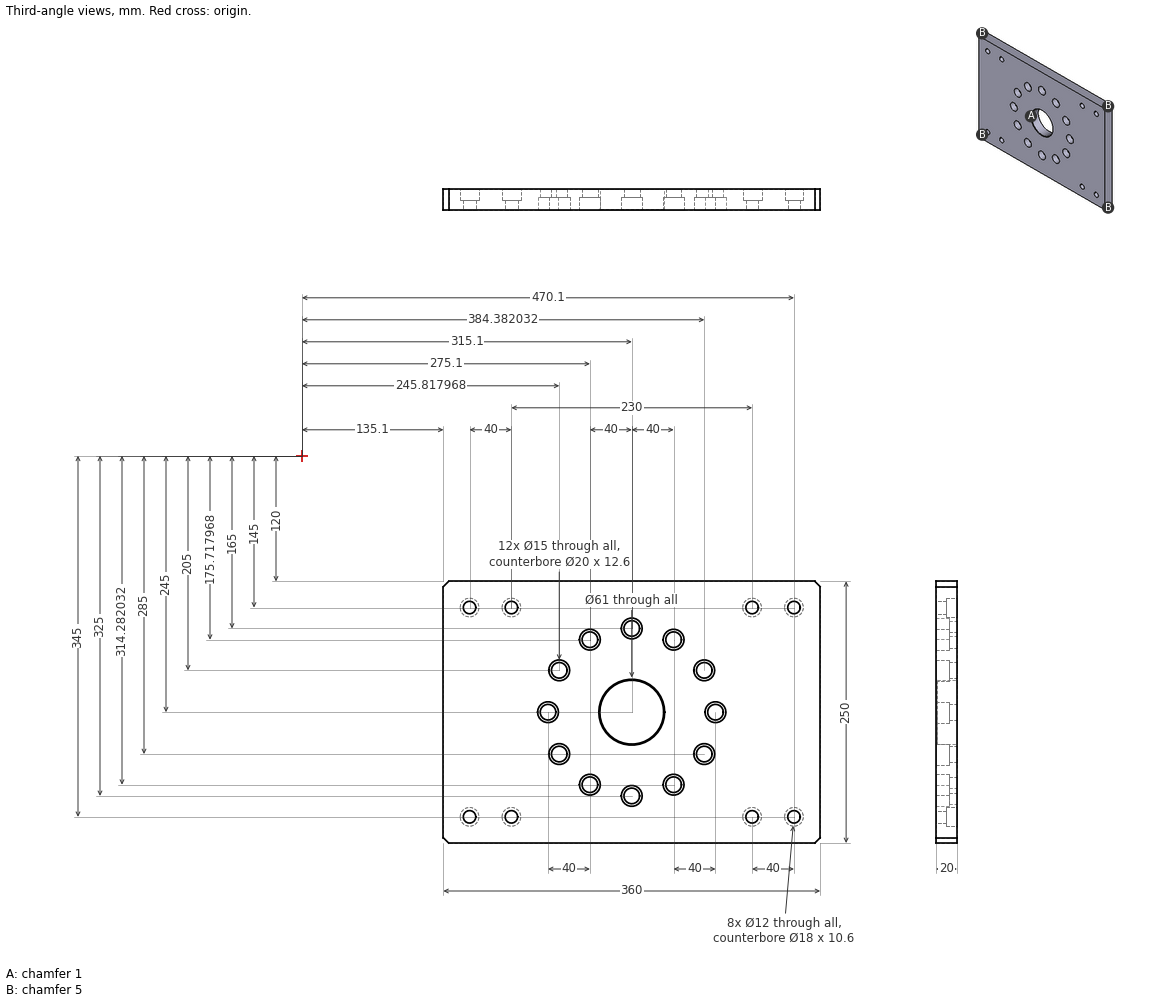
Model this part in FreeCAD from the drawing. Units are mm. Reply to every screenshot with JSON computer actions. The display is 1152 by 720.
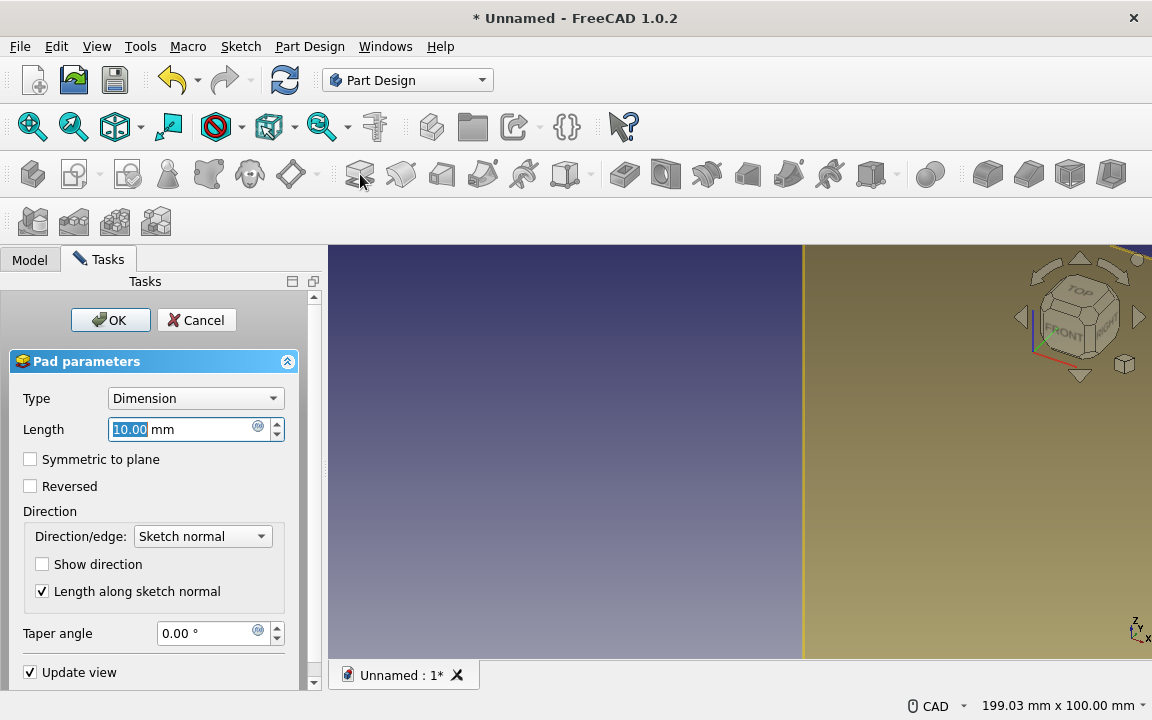
{"action": "type", "text": "20"}
{"action": "key", "text": "Tab"}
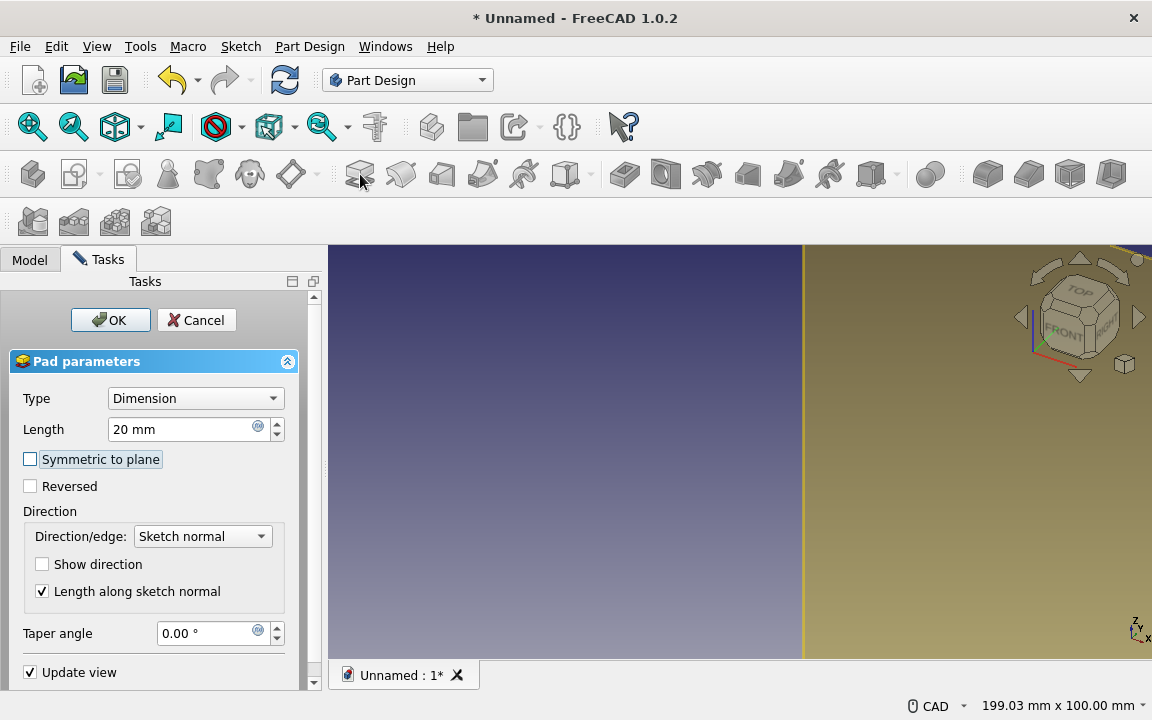
{"action": "left_click", "coordinate": [31, 486]}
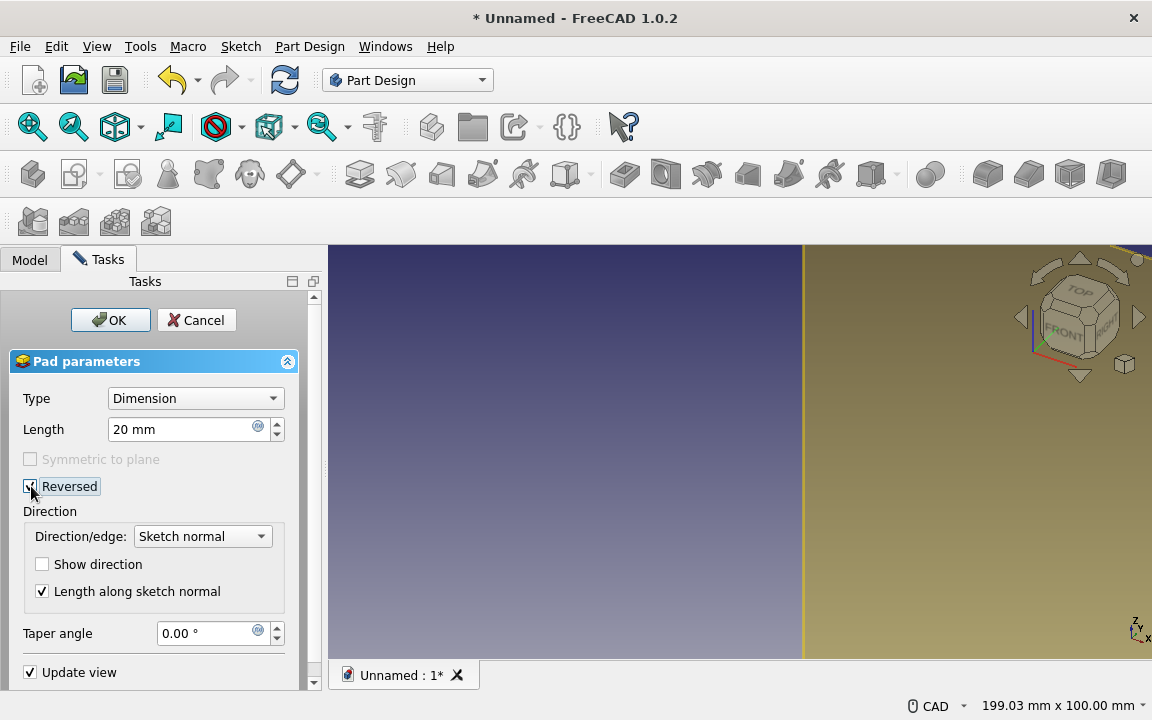
{"action": "left_click", "coordinate": [111, 320]}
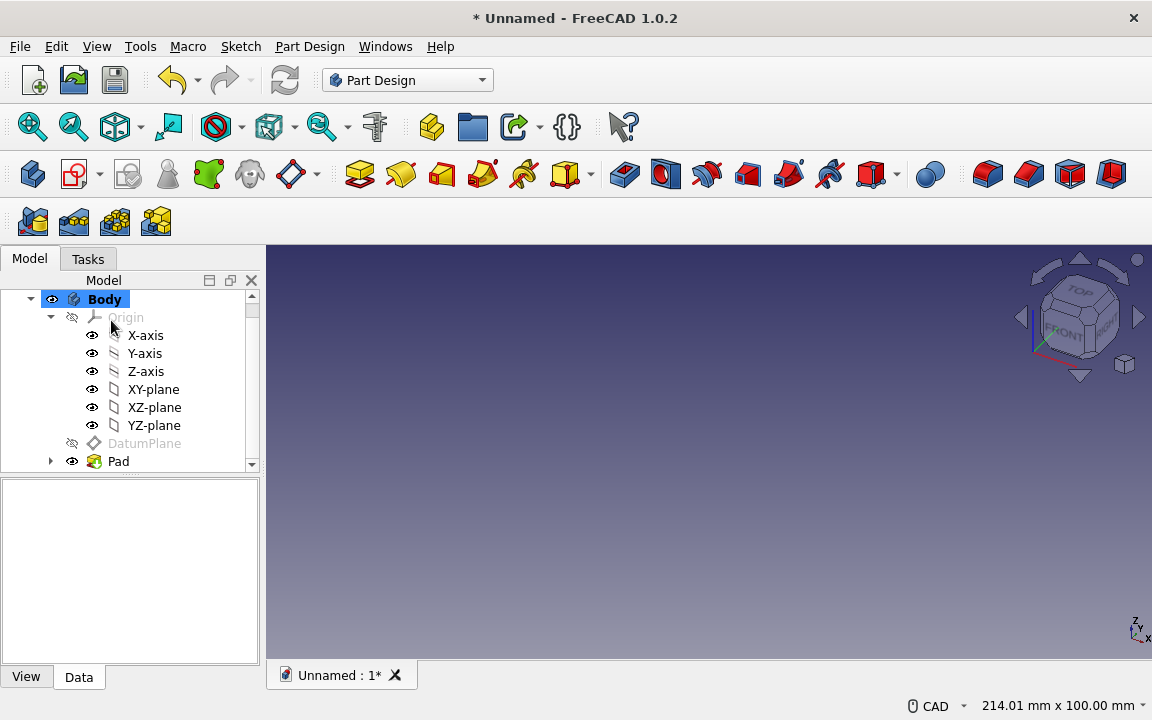
{"action": "left_click", "coordinate": [33, 128]}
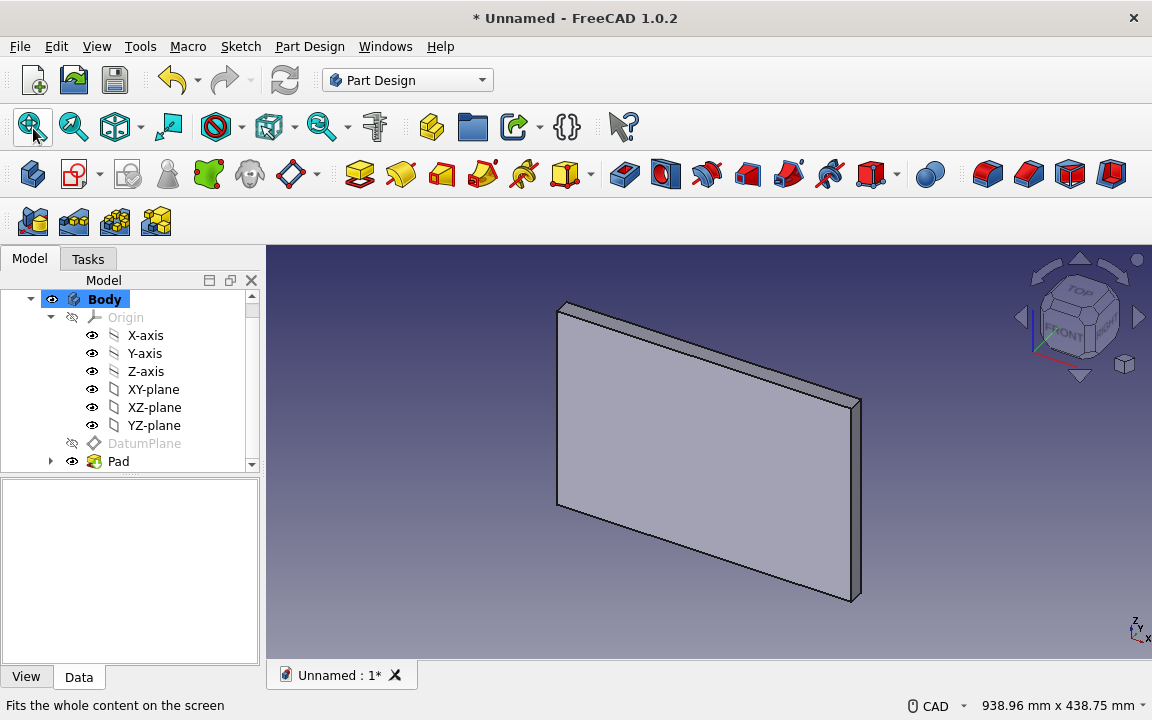
{"action": "key", "text": "4"}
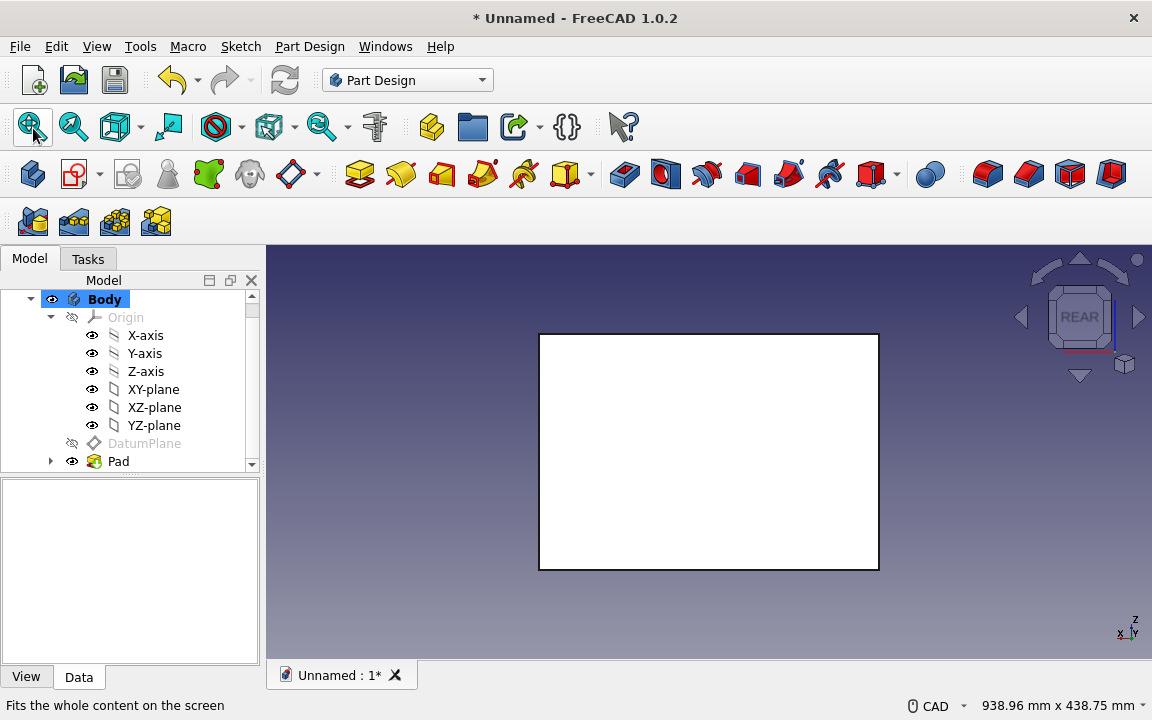
{"action": "left_click", "coordinate": [660, 451]}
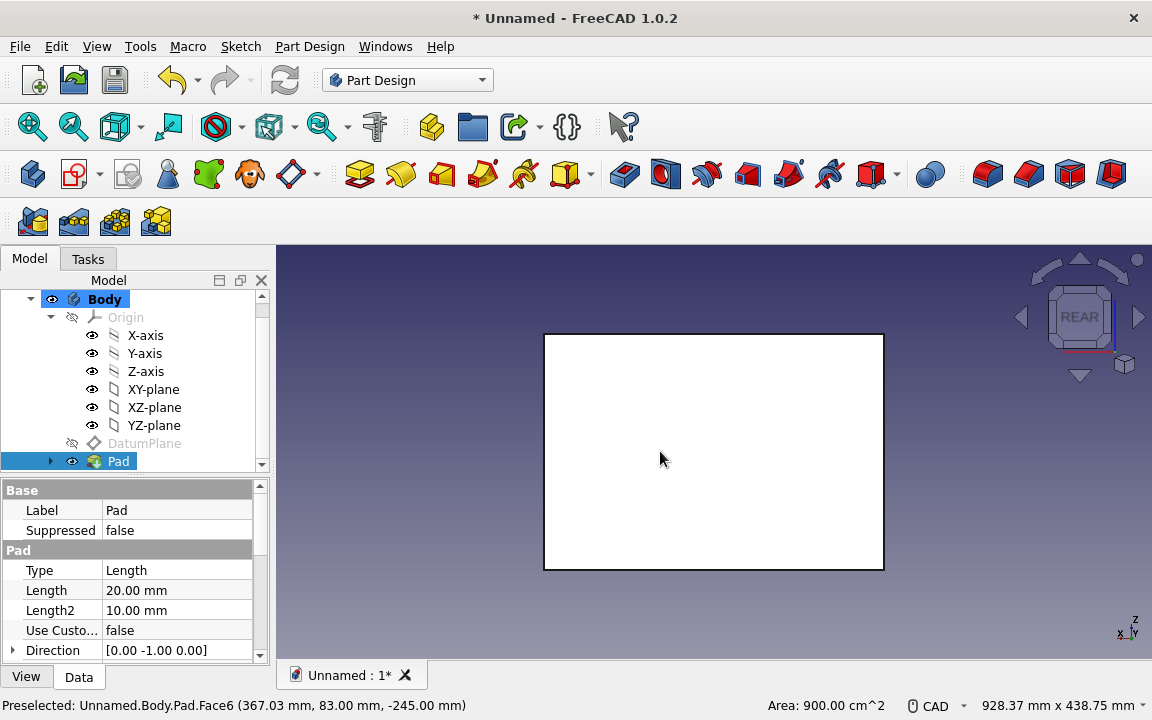
{"action": "left_click", "coordinate": [74, 174]}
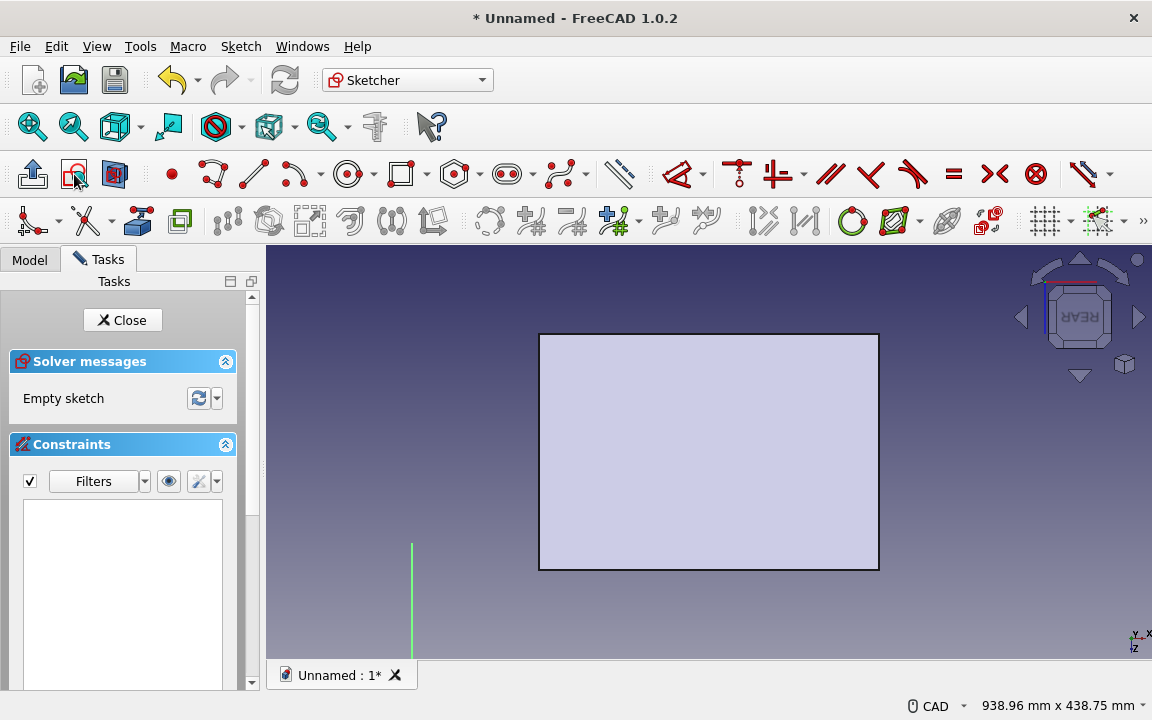
{"action": "scroll", "coordinate": [649, 319], "scroll_direction": "down", "scroll_amount": 2}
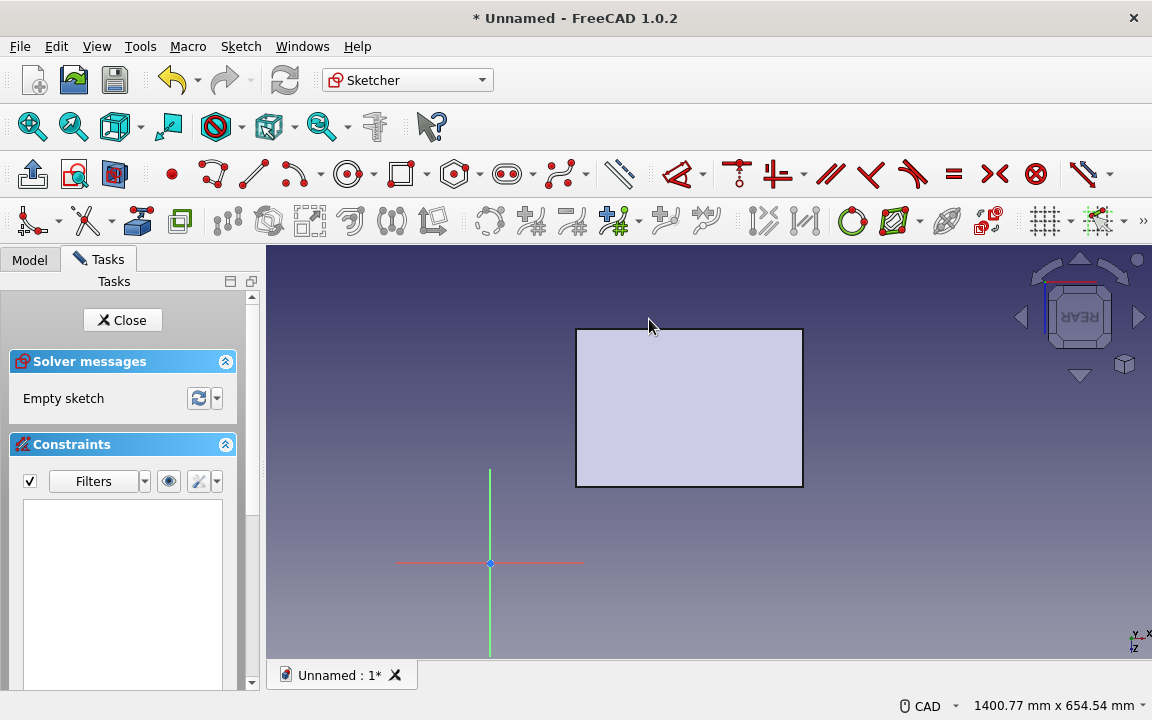
{"action": "left_click", "coordinate": [348, 174]}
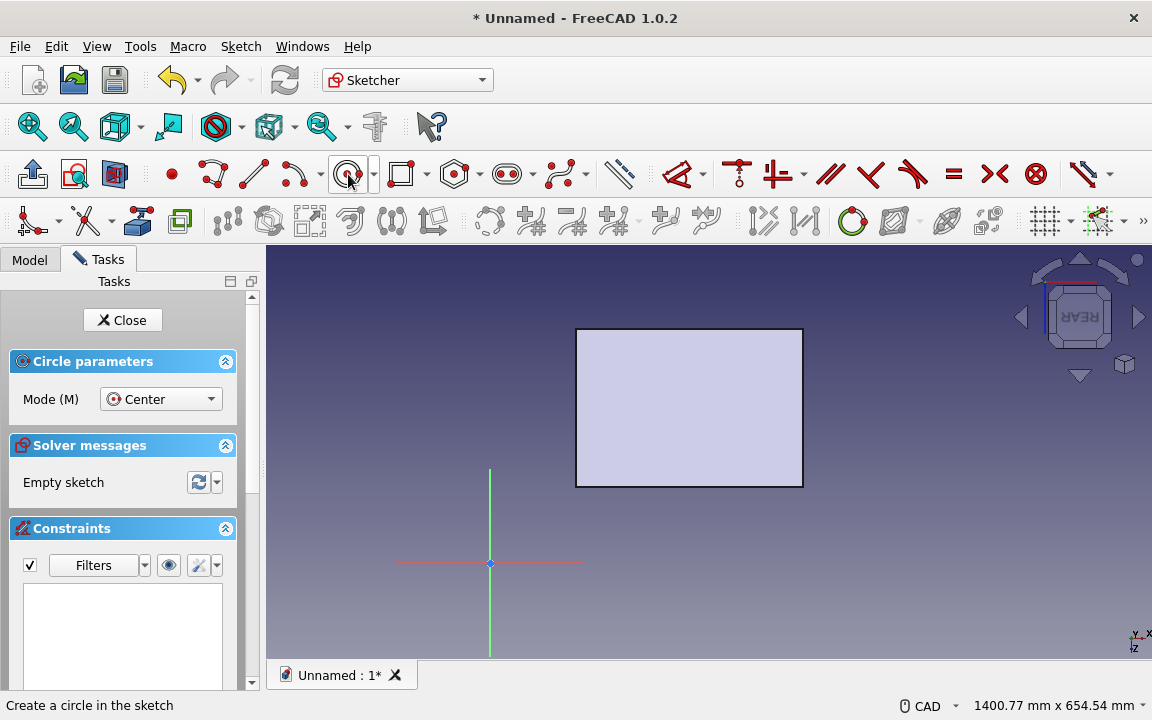
{"action": "scroll", "coordinate": [787, 345], "scroll_direction": "up", "scroll_amount": 9}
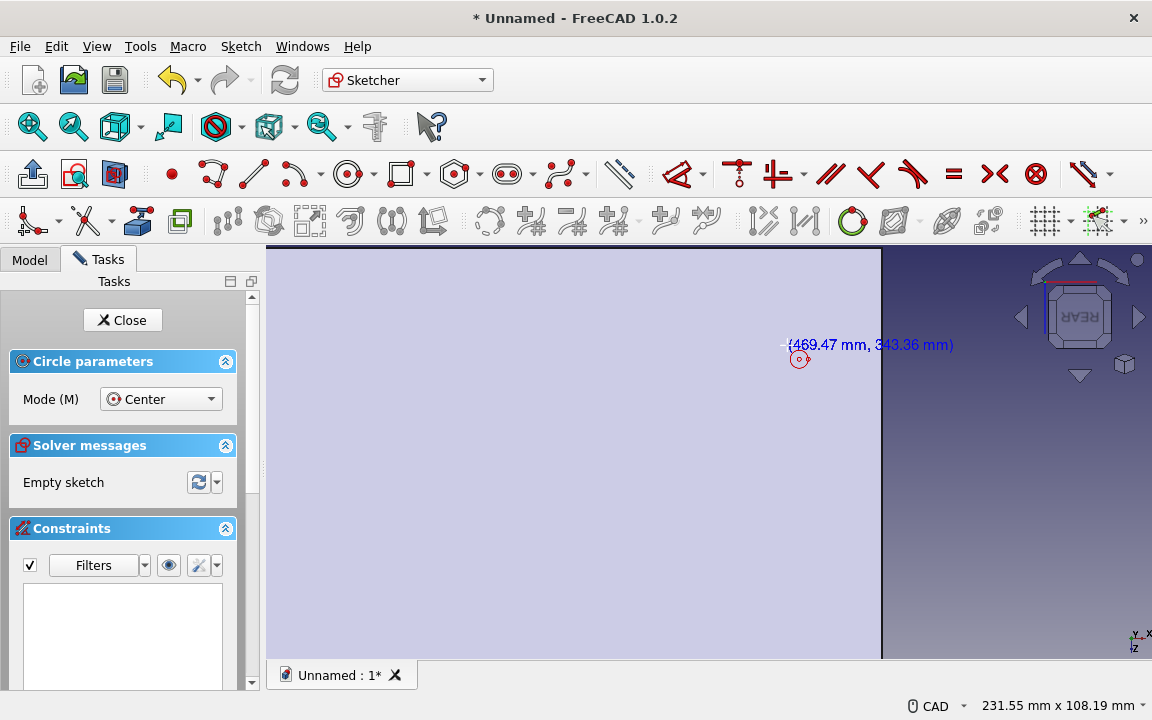
{"action": "scroll", "coordinate": [828, 315], "scroll_direction": "down", "scroll_amount": 8}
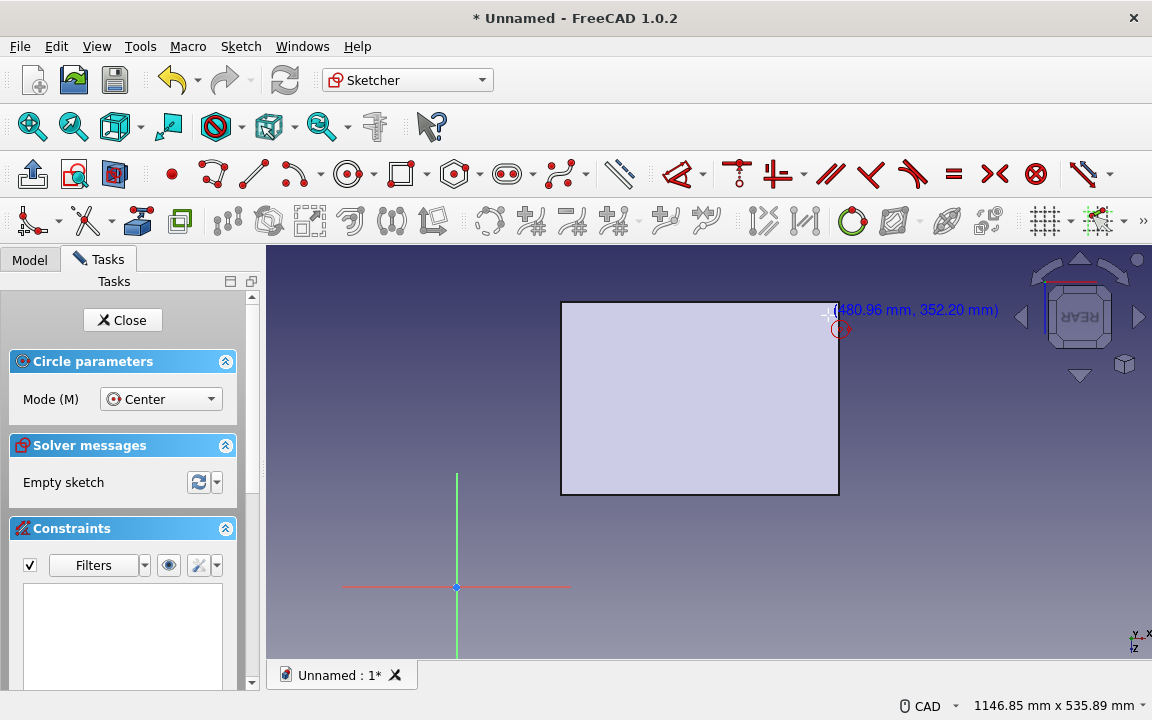
{"action": "left_click", "coordinate": [820, 321]}
{"action": "mouse_move", "coordinate": [823, 318]}